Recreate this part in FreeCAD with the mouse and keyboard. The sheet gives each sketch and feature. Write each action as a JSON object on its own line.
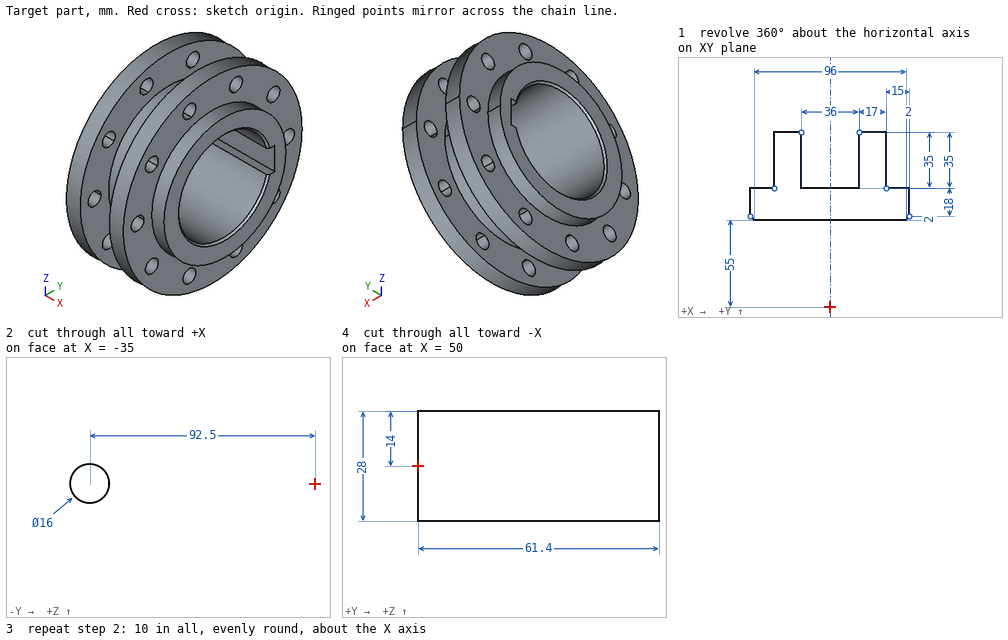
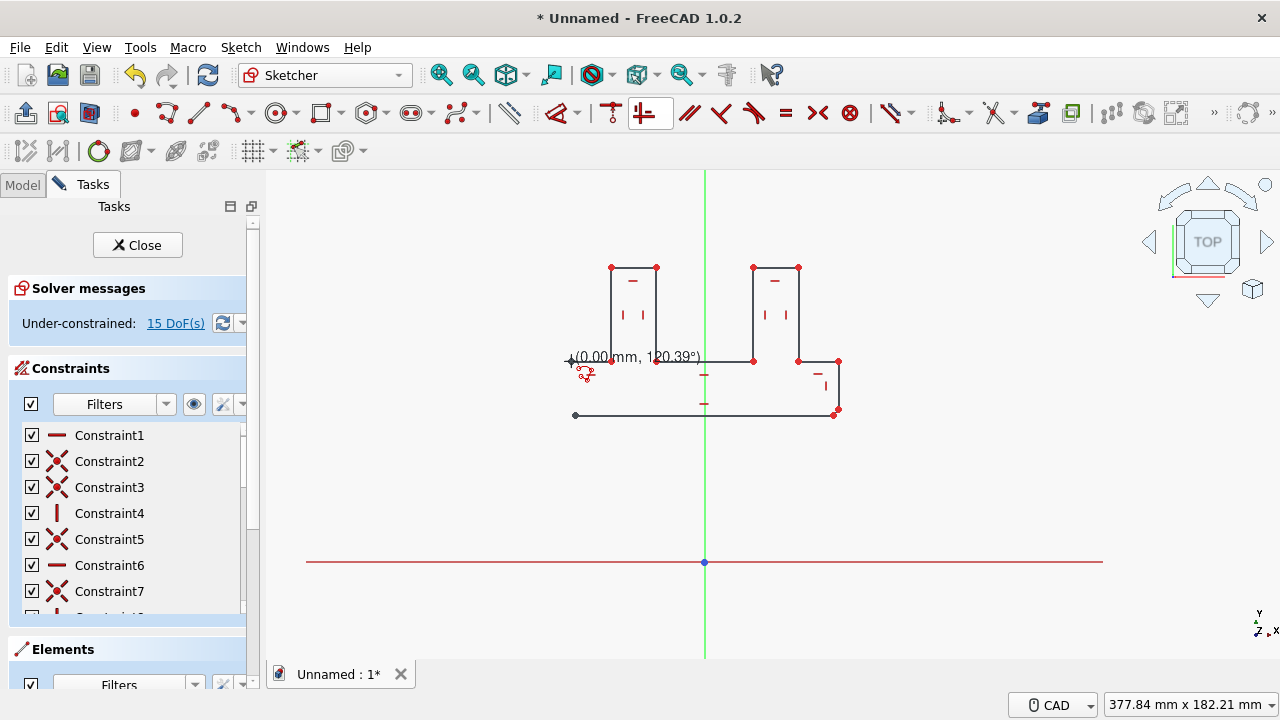
{"action": "scroll", "coordinate": [571, 409], "scroll_direction": "up", "scroll_amount": 4}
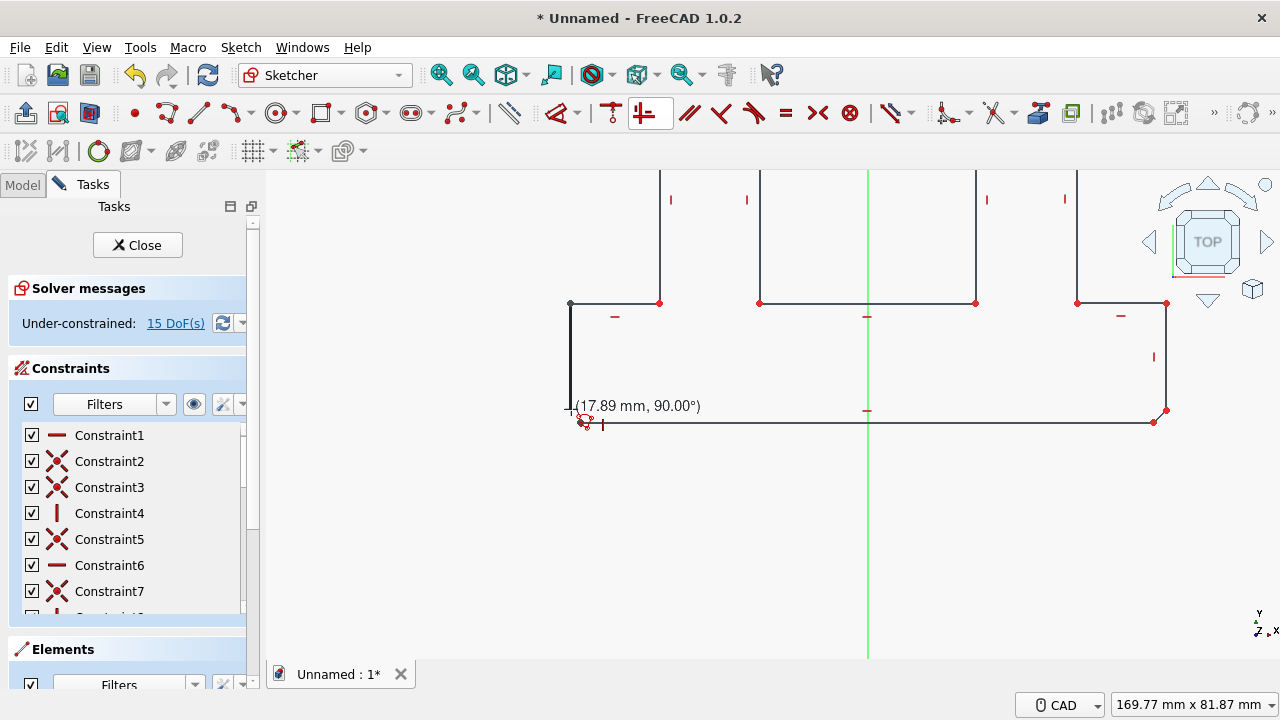
{"action": "left_click", "coordinate": [571, 409]}
{"action": "left_click", "coordinate": [580, 423]}
{"action": "key", "text": "Escape"}
{"action": "key", "text": "Escape"}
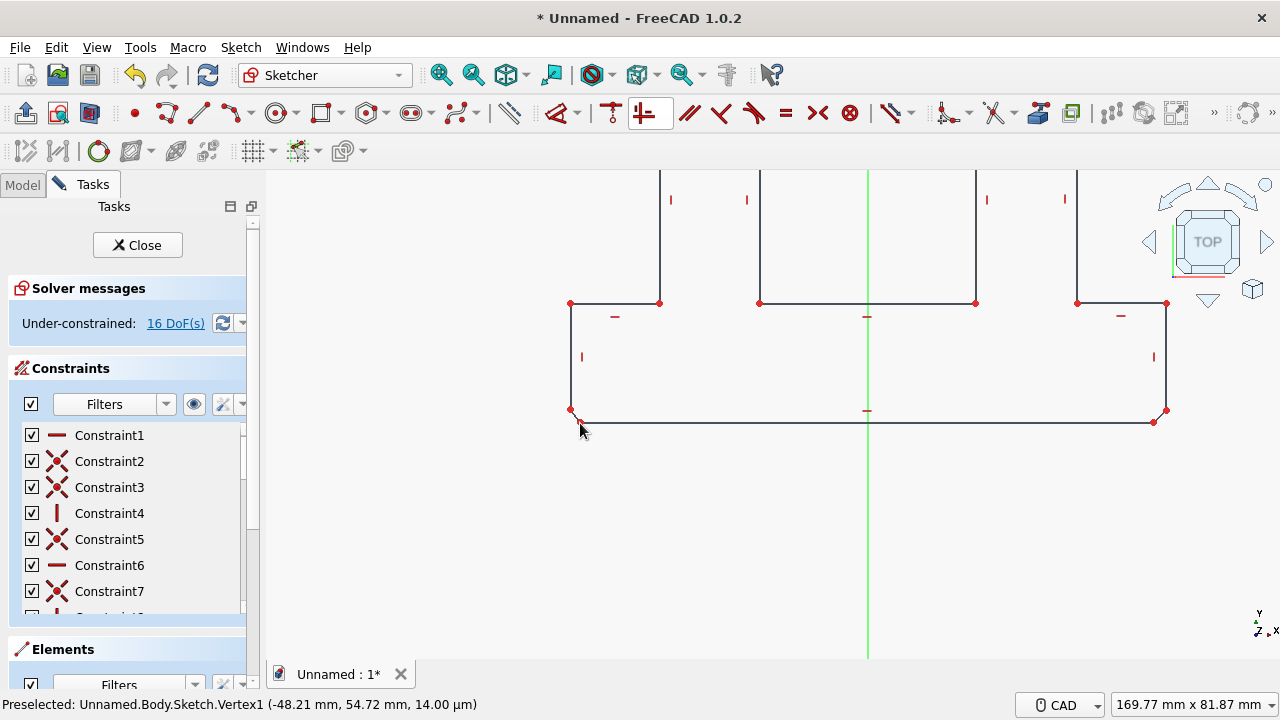
{"action": "scroll", "coordinate": [571, 409], "scroll_direction": "down", "scroll_amount": 4}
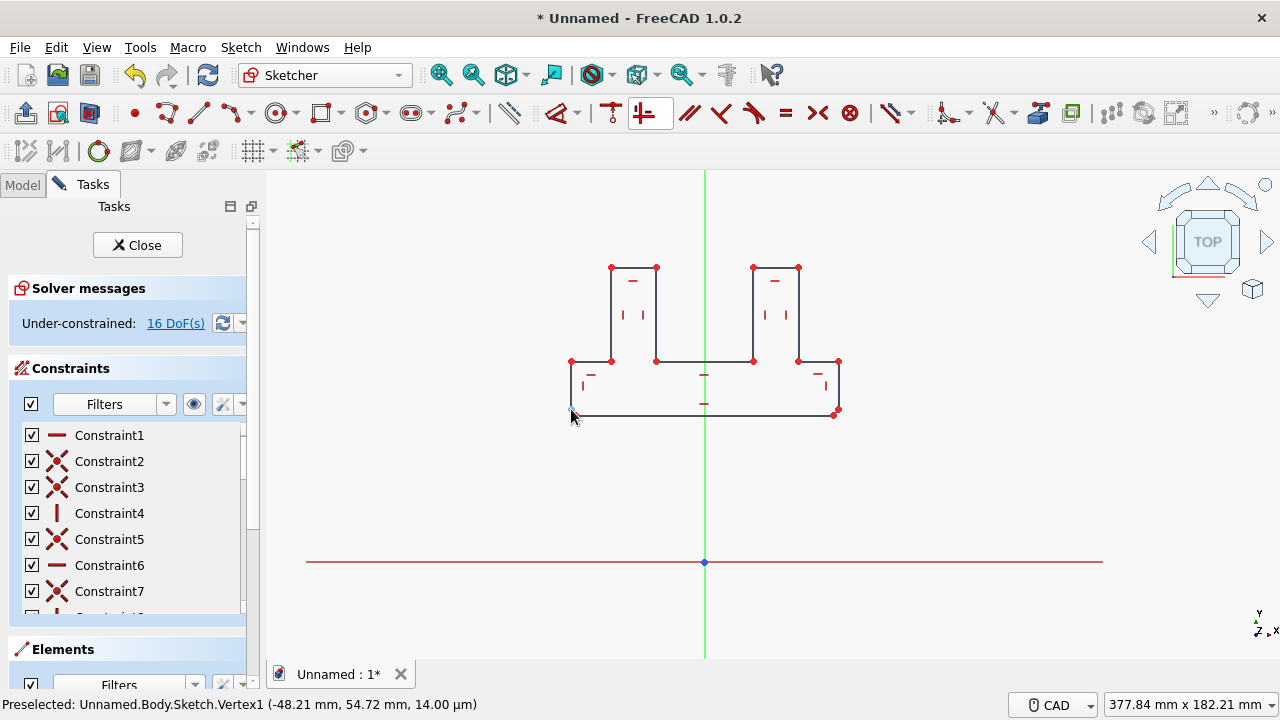
{"action": "left_click", "coordinate": [753, 268]}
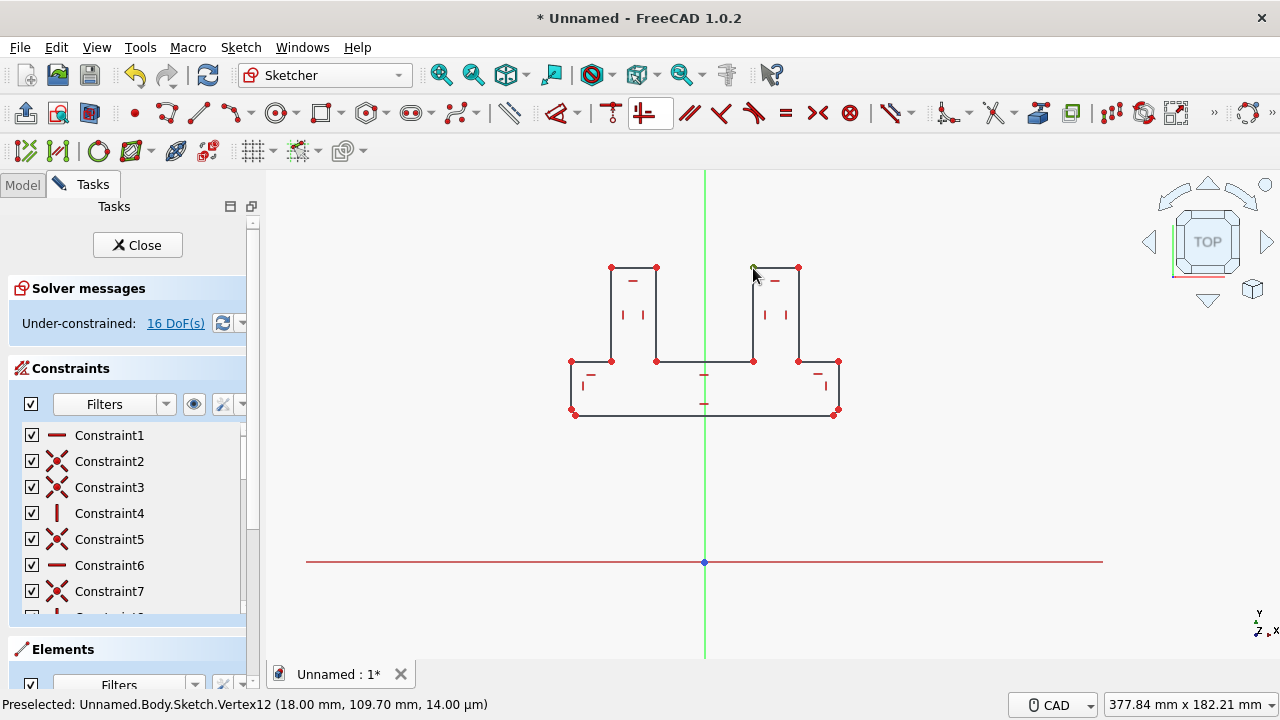
{"action": "left_click", "coordinate": [656, 268]}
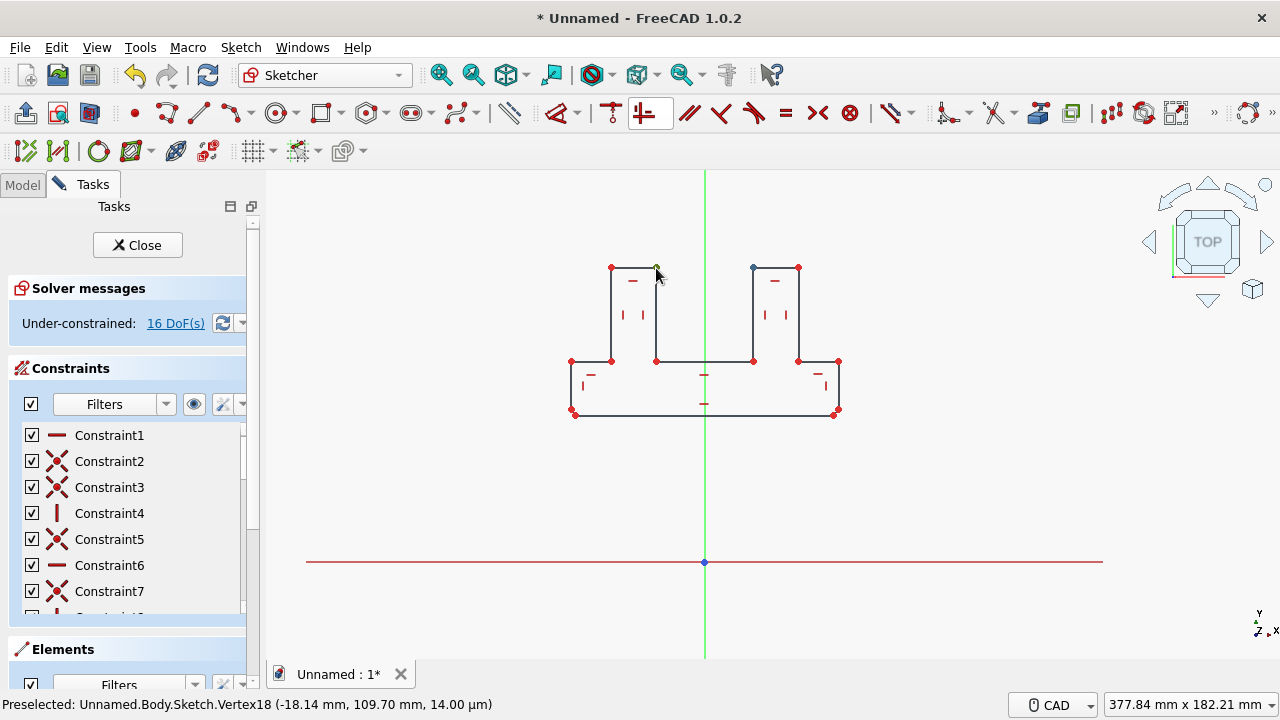
{"action": "left_click", "coordinate": [705, 600]}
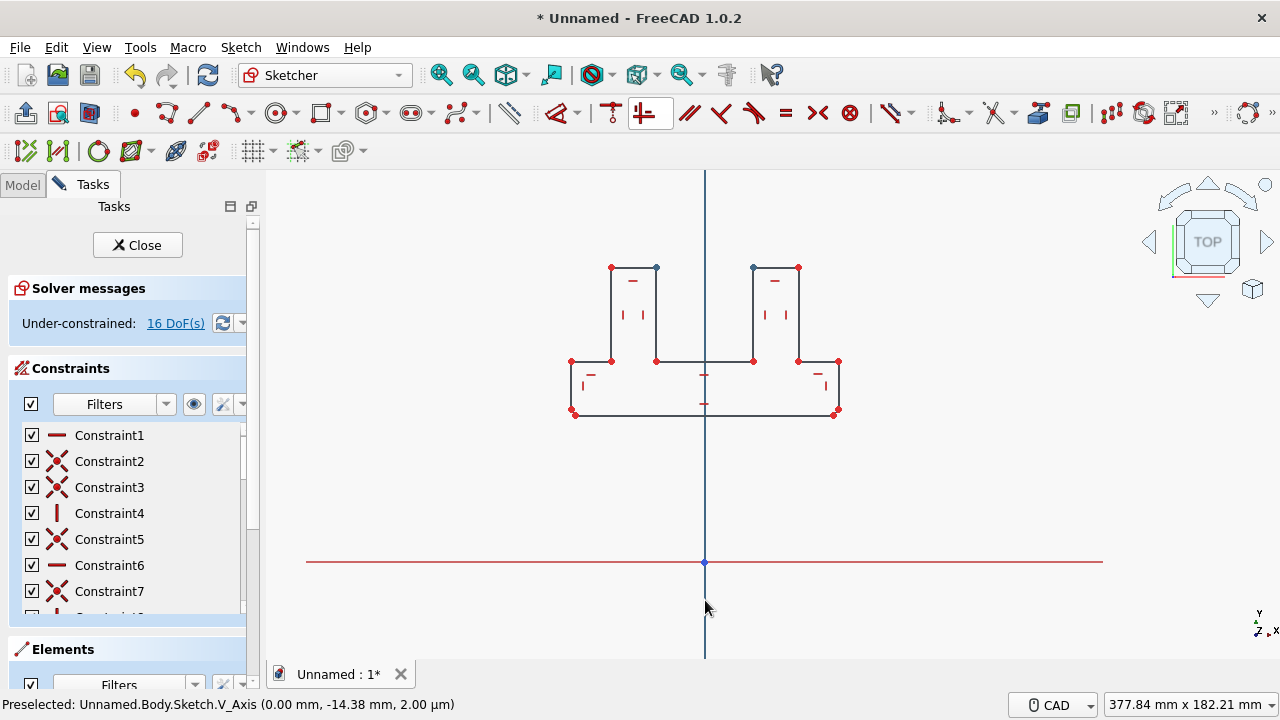
{"action": "left_click", "coordinate": [818, 114]}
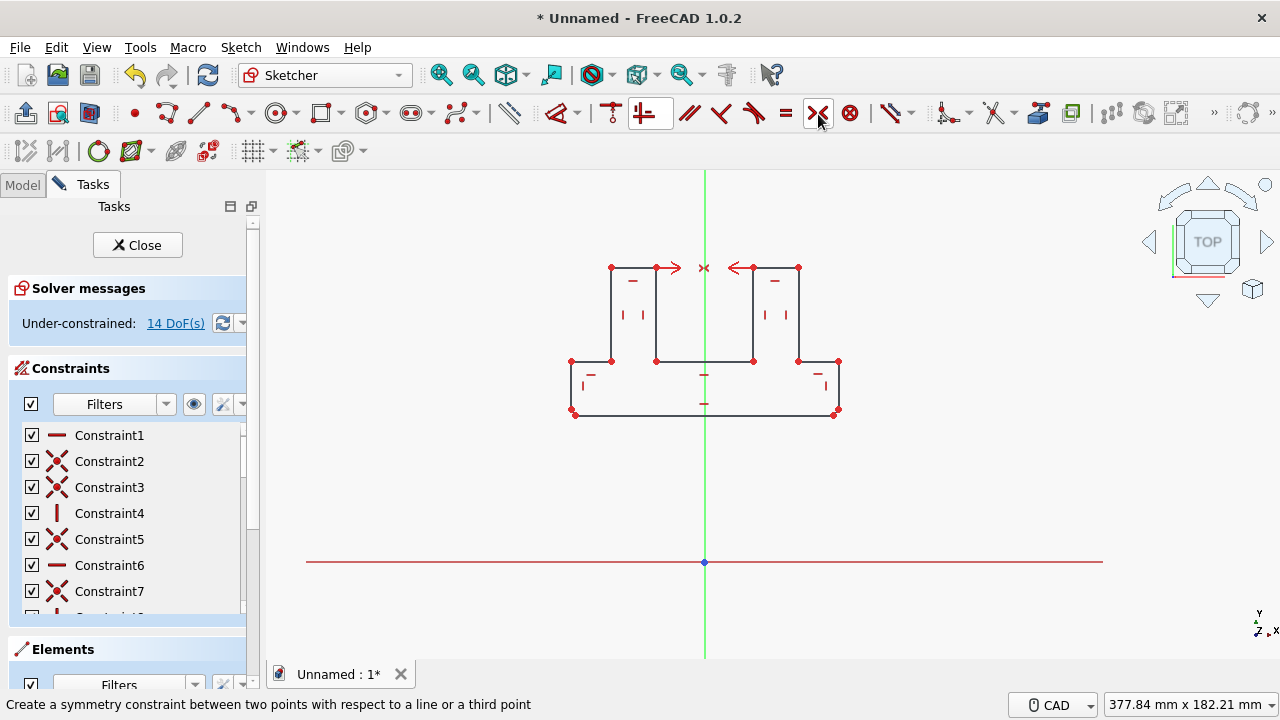
{"action": "left_click", "coordinate": [799, 362]}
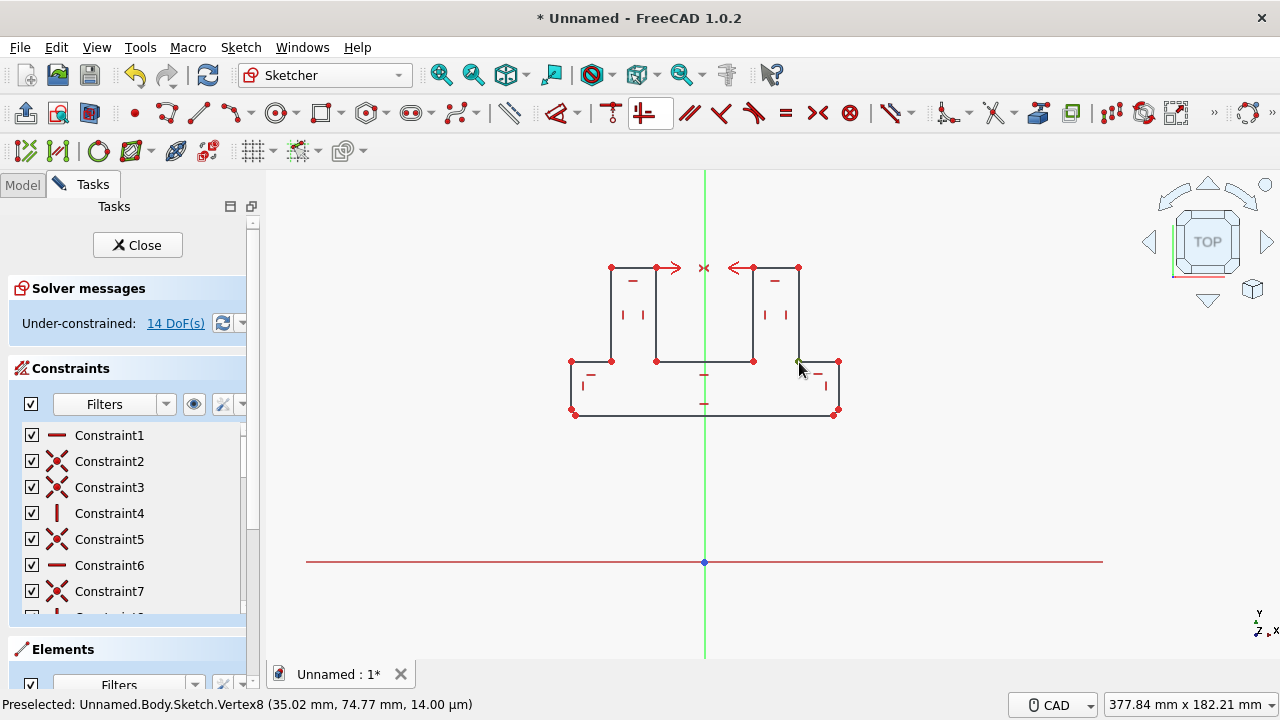
{"action": "left_click", "coordinate": [611, 362]}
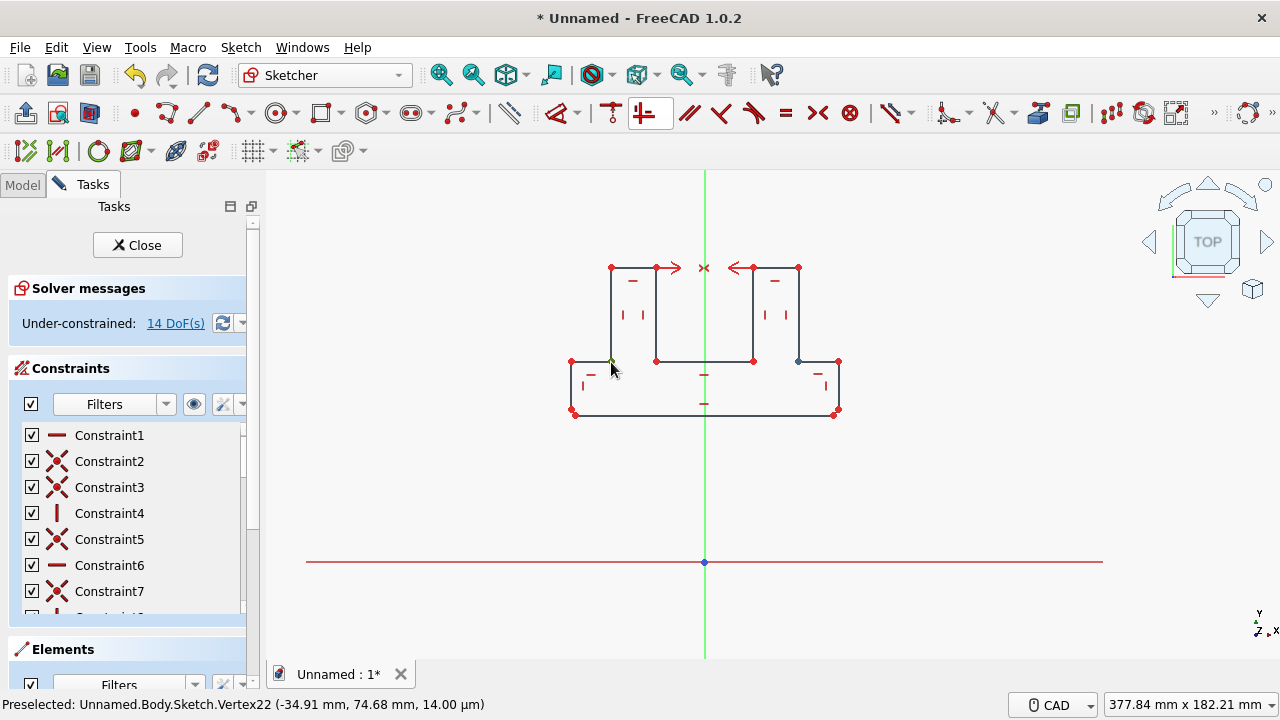
{"action": "left_click", "coordinate": [705, 600]}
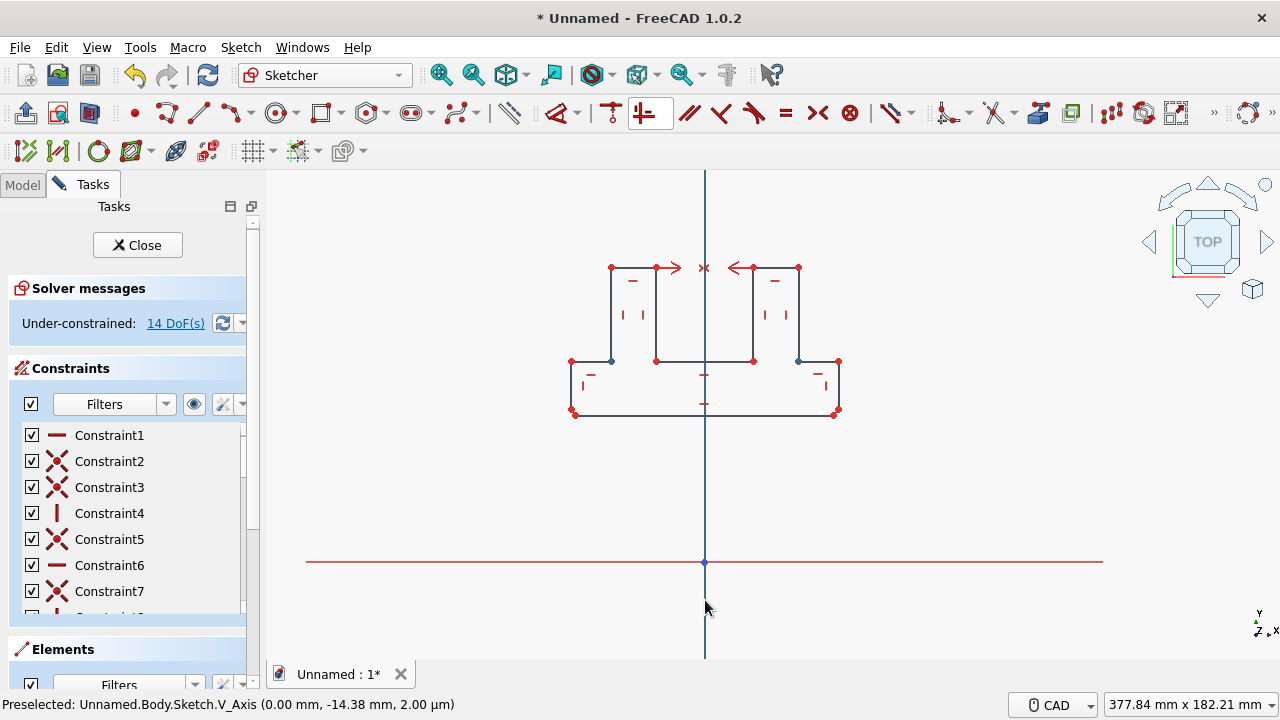
{"action": "left_click", "coordinate": [818, 114]}